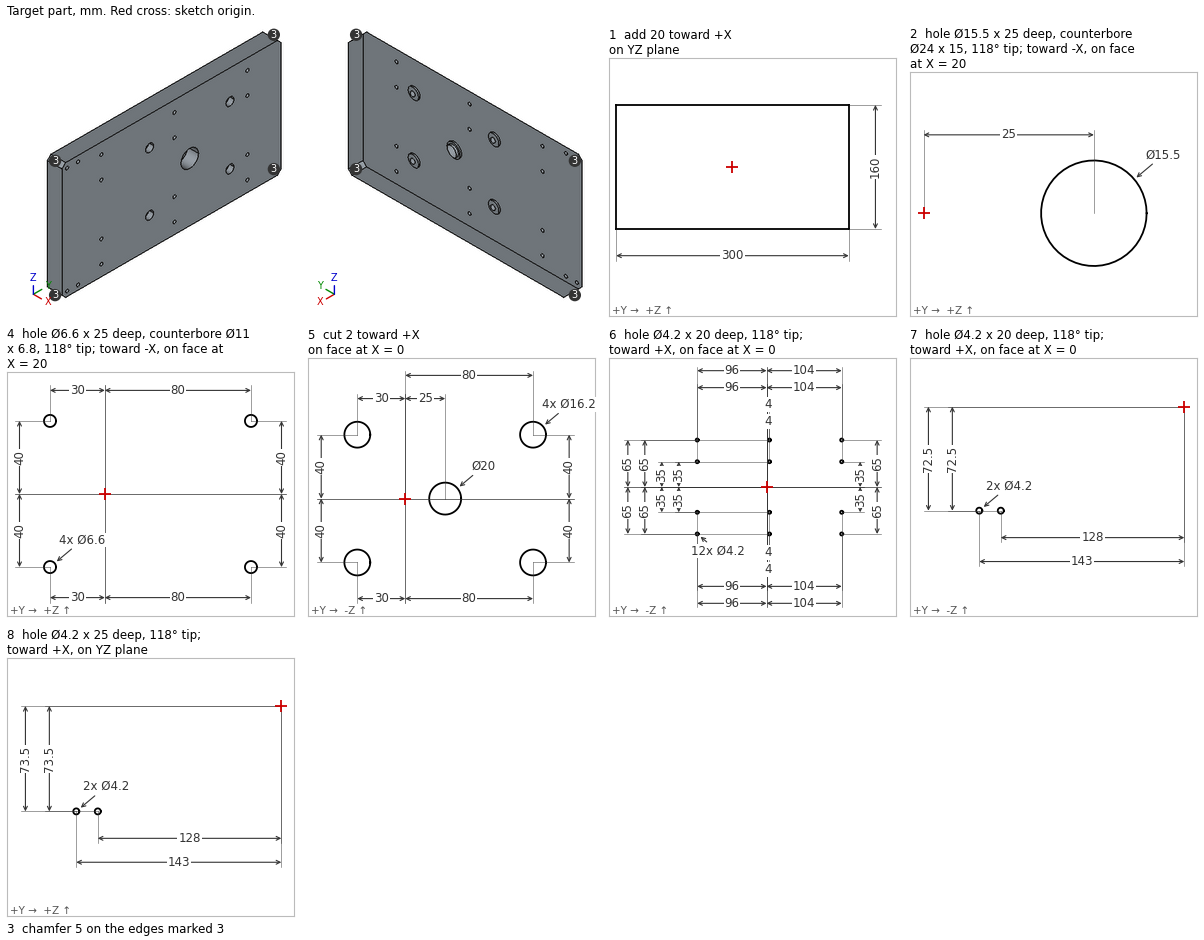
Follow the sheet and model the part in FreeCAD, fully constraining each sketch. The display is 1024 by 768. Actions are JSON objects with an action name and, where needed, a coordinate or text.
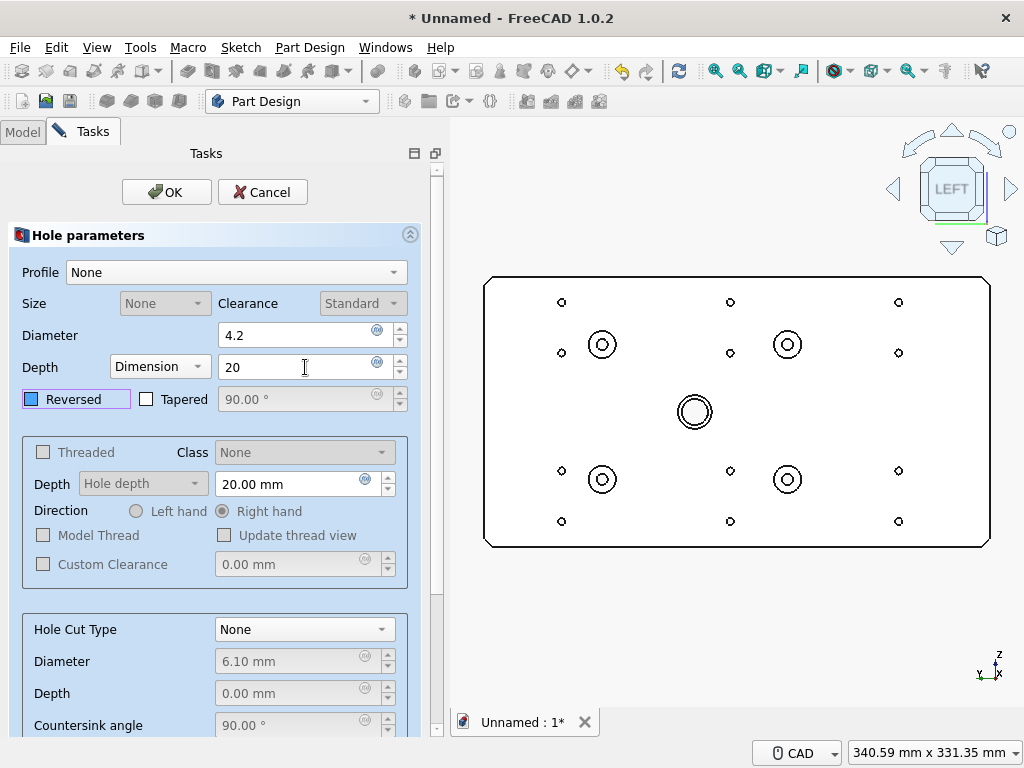
{"action": "left_click", "coordinate": [167, 192]}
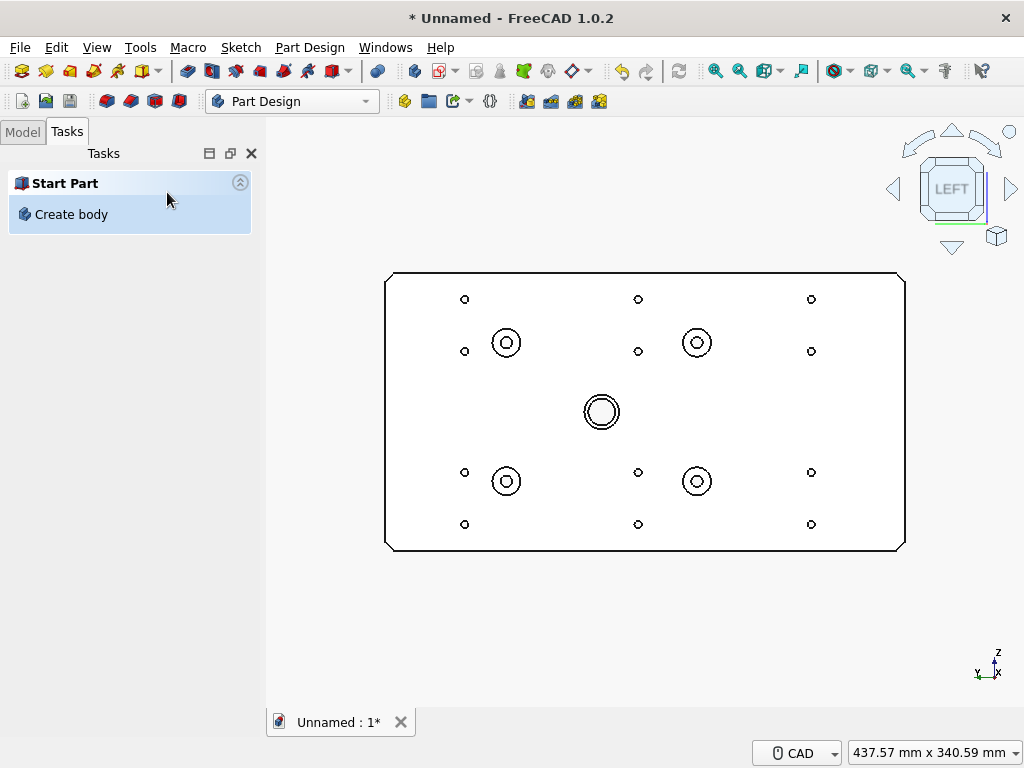
{"action": "left_click", "coordinate": [793, 411]}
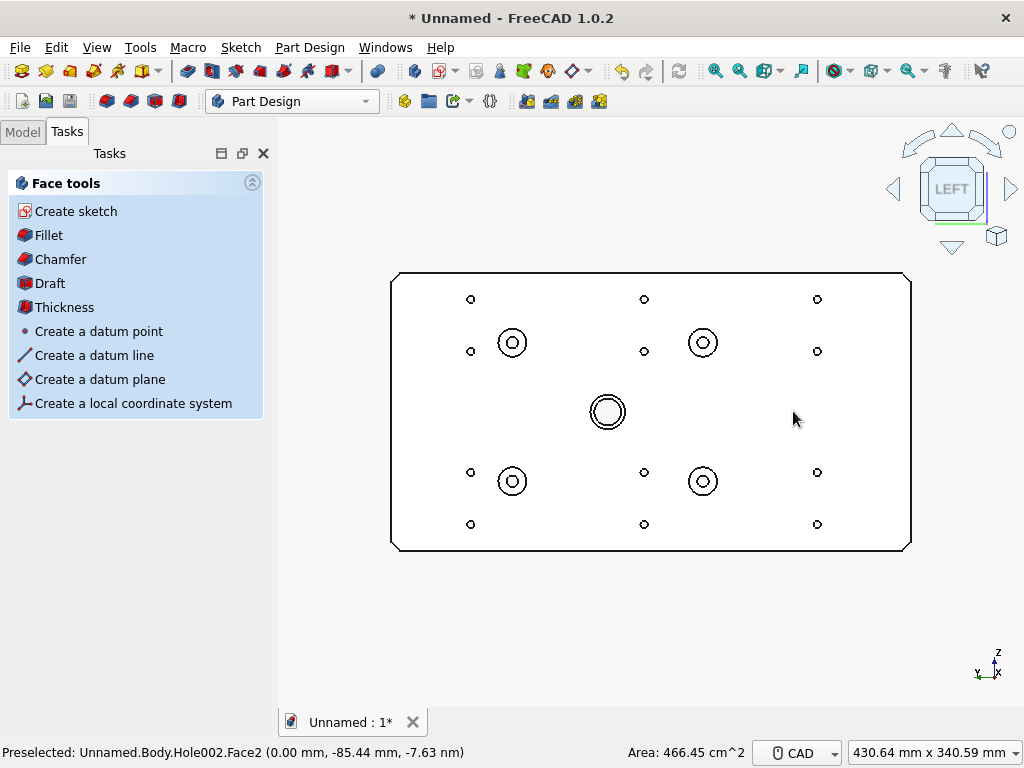
{"action": "left_click", "coordinate": [440, 72]}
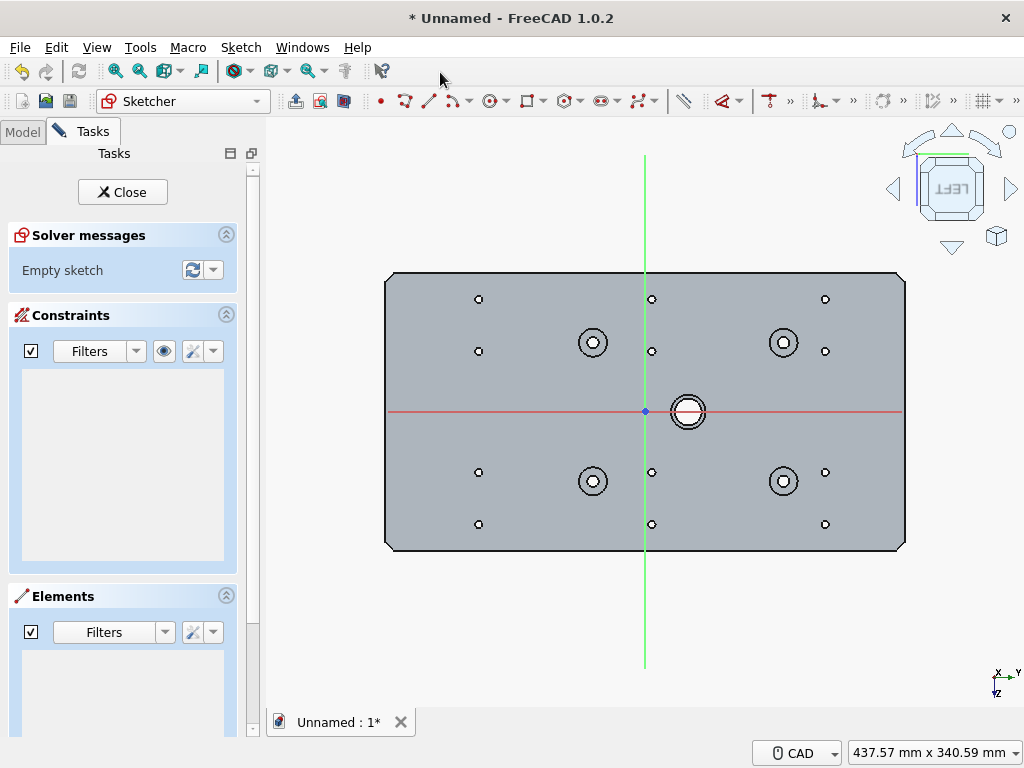
{"action": "scroll", "coordinate": [394, 550], "scroll_direction": "up", "scroll_amount": 12}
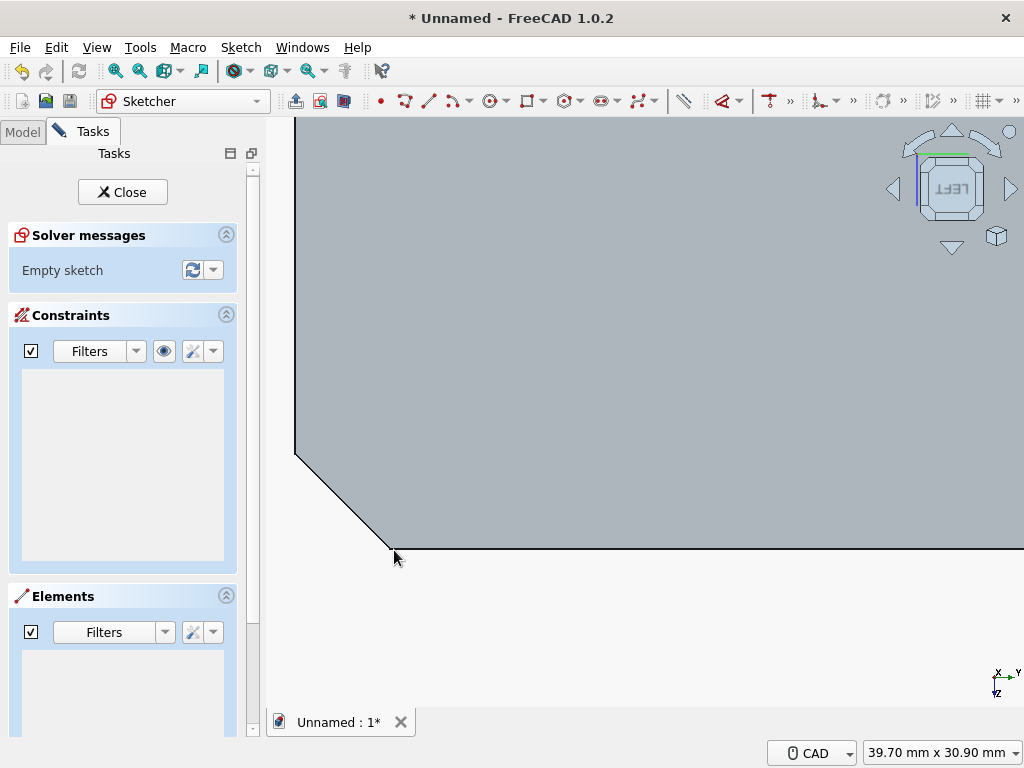
{"action": "left_click", "coordinate": [490, 102]}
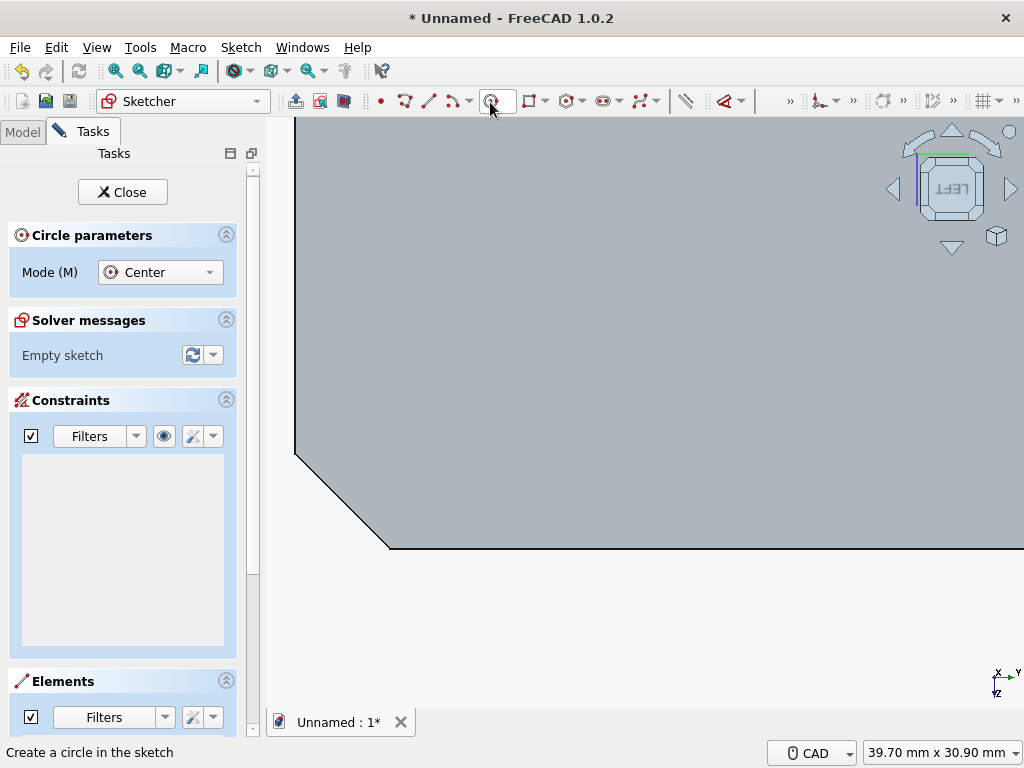
{"action": "left_click", "coordinate": [428, 406]}
{"action": "left_click", "coordinate": [457, 377]}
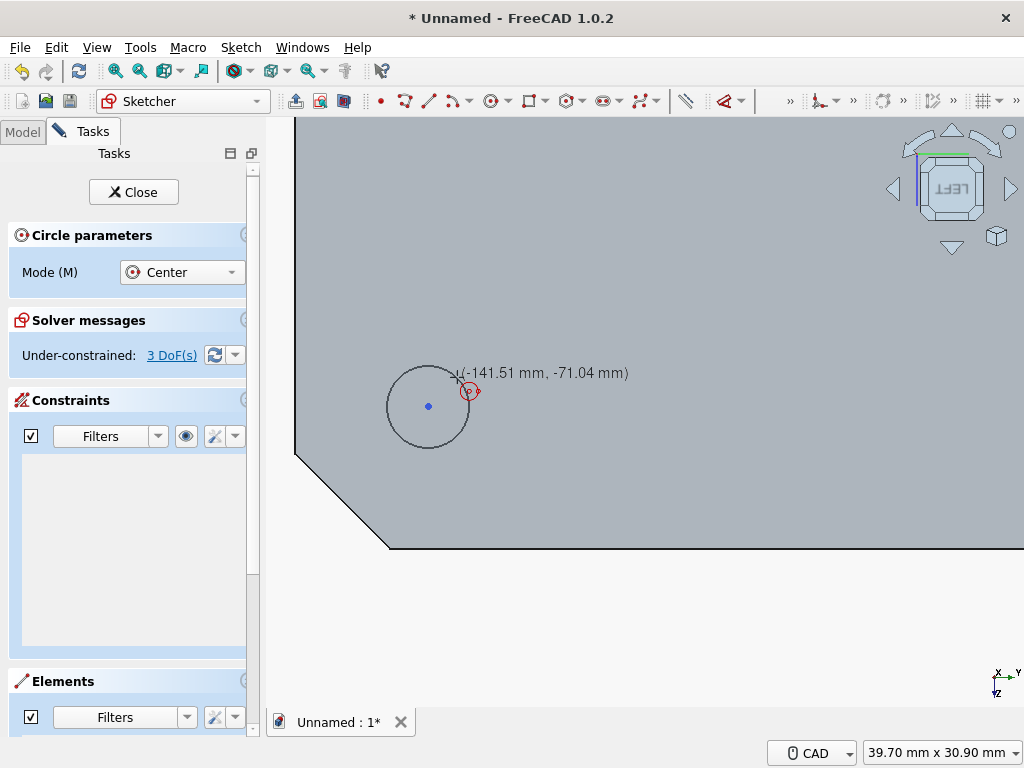
{"action": "left_click", "coordinate": [715, 406]}
{"action": "left_click", "coordinate": [743, 377]}
{"action": "key", "text": "Escape"}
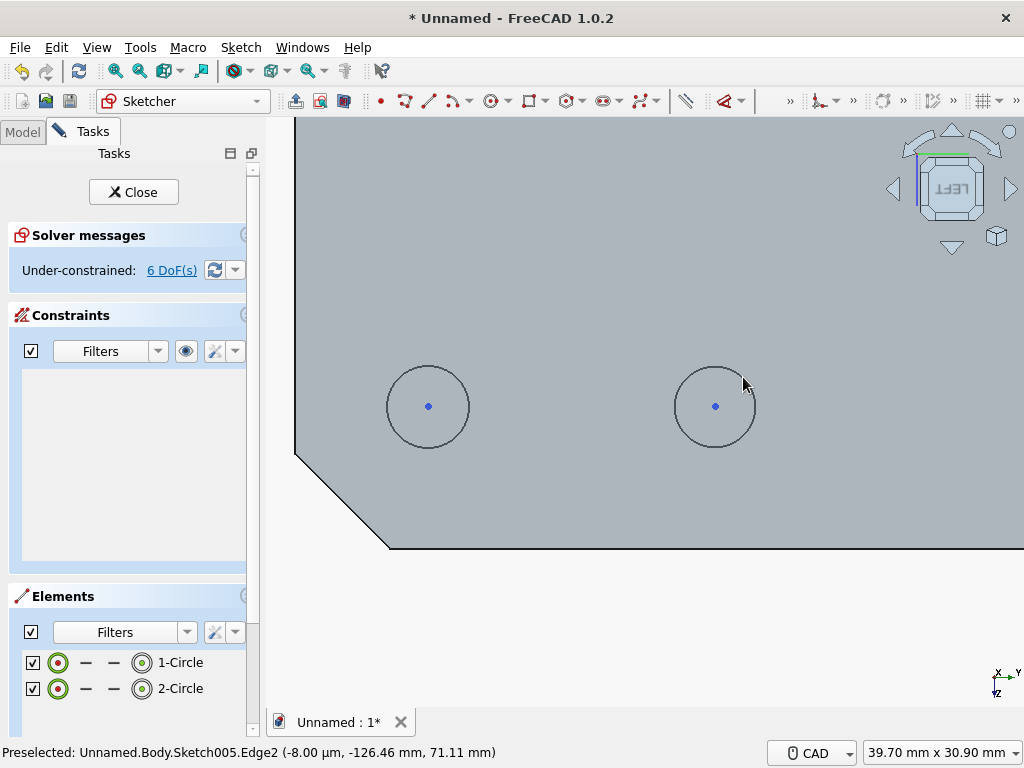
{"action": "left_click", "coordinate": [457, 378]}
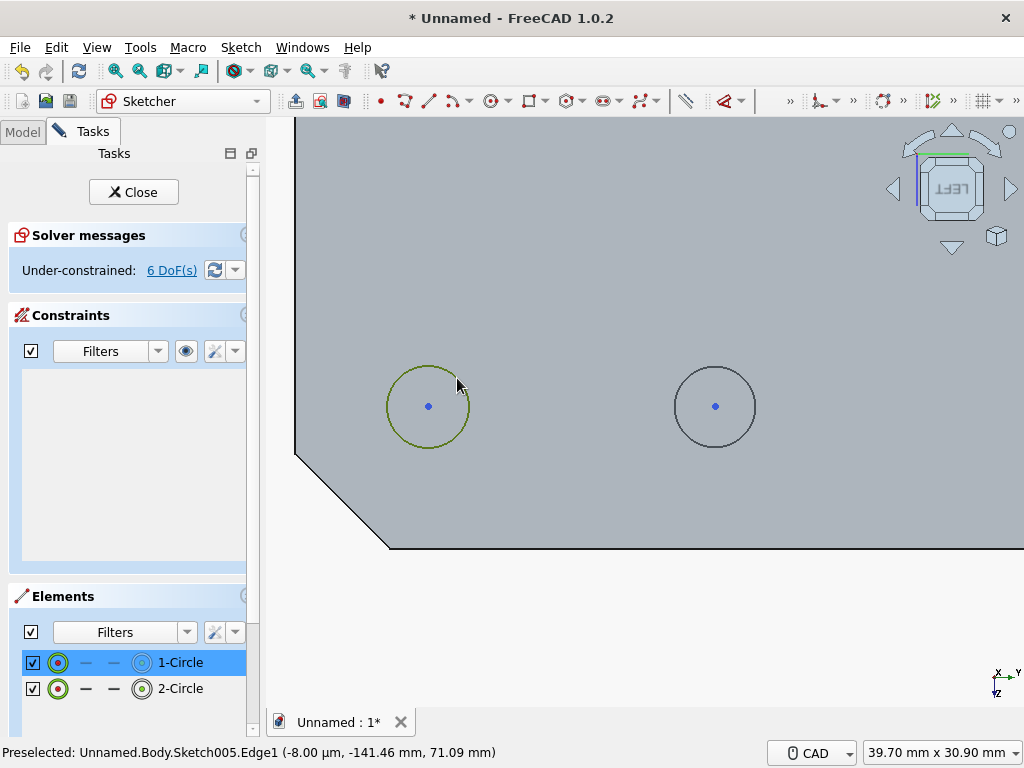
{"action": "left_click", "coordinate": [743, 378]}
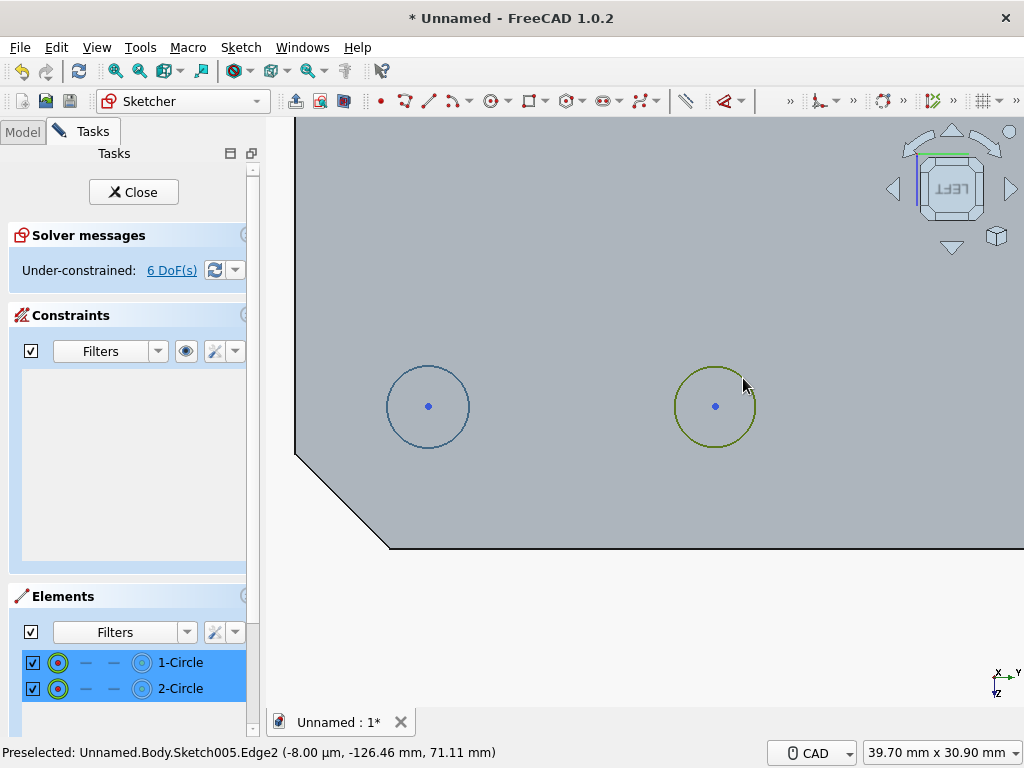
{"action": "key", "text": "e"}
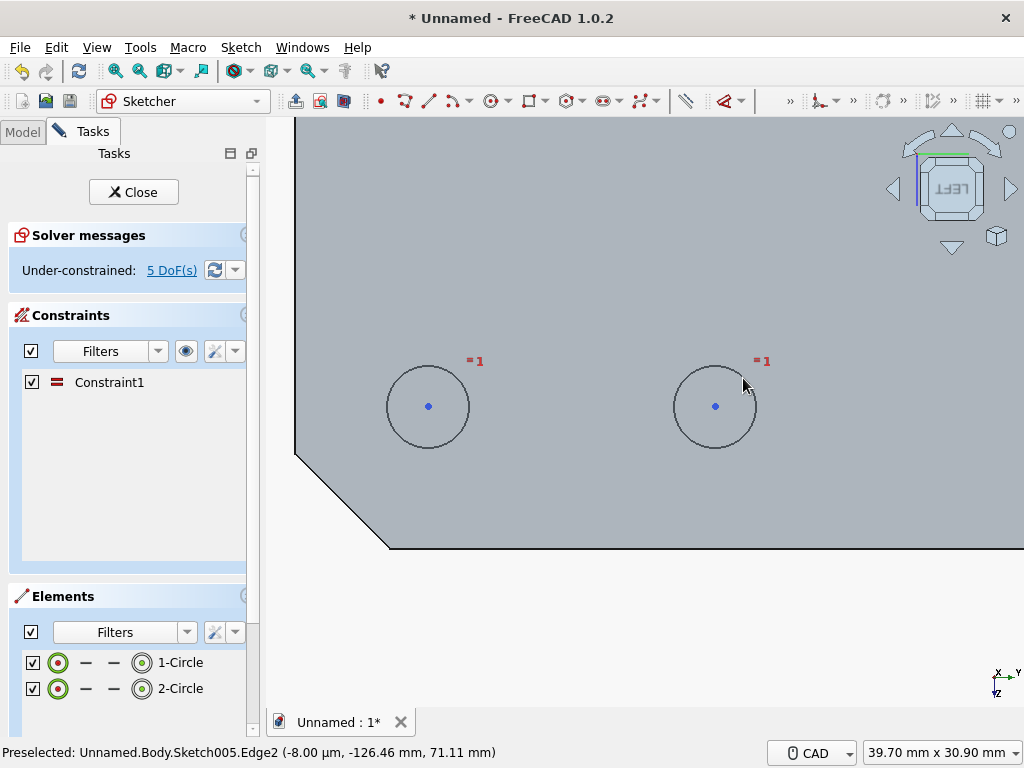
{"action": "key", "text": "d"}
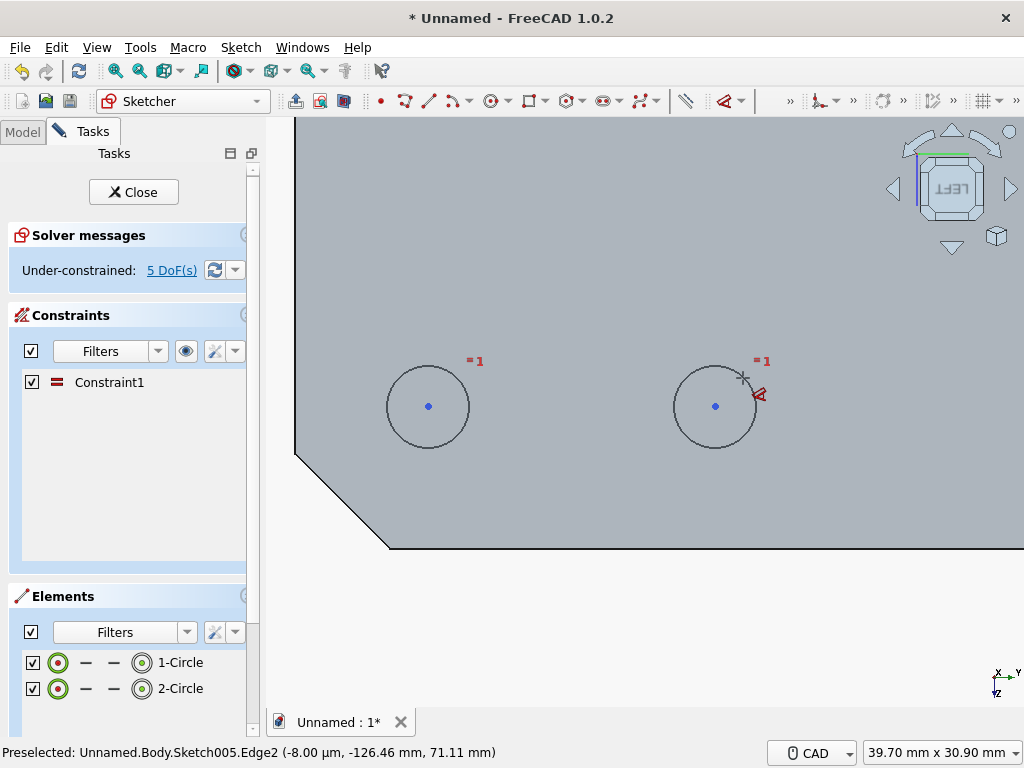
{"action": "left_click", "coordinate": [457, 378]}
{"action": "left_click", "coordinate": [480, 355]}